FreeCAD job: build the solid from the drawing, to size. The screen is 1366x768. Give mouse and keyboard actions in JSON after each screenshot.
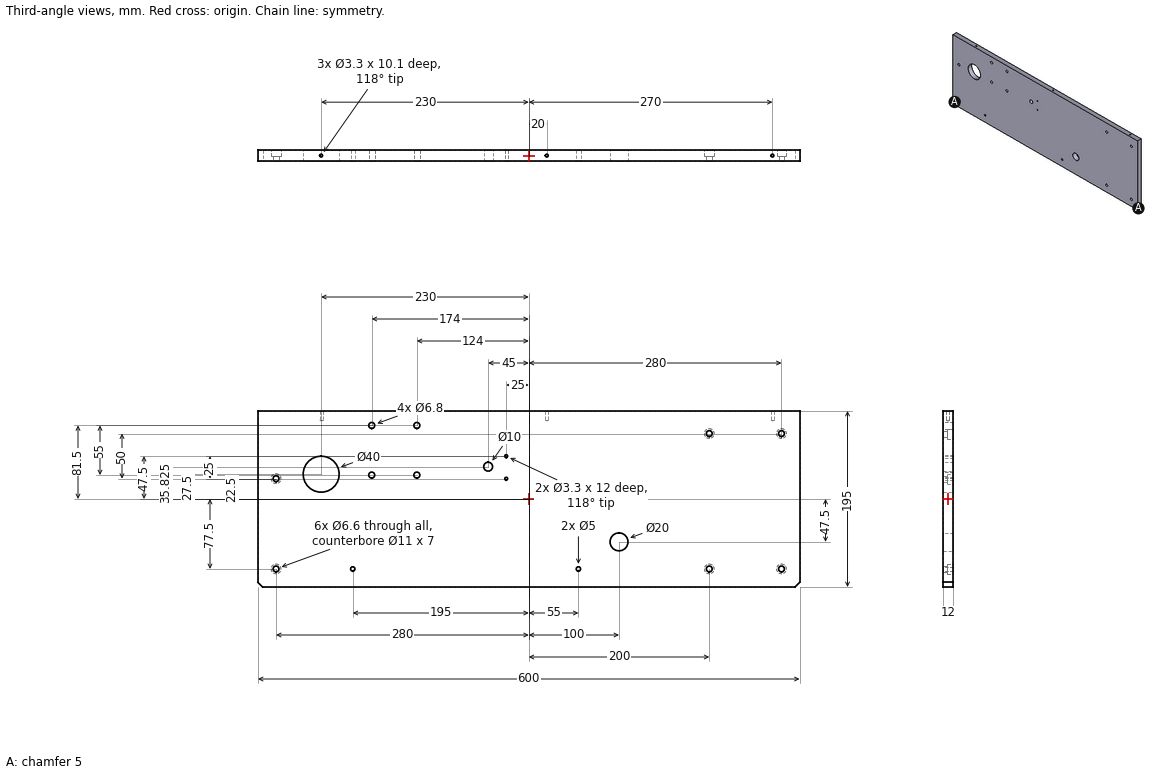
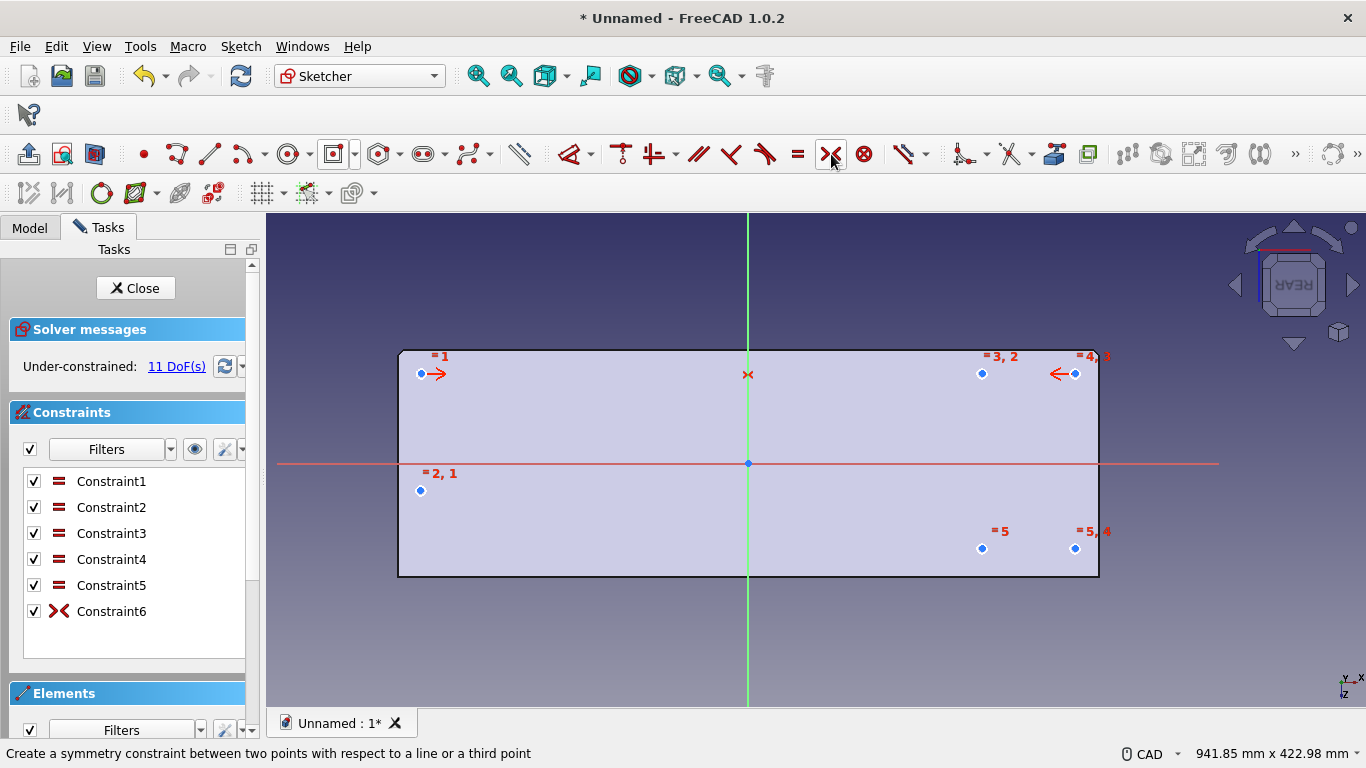
{"action": "key", "text": "d"}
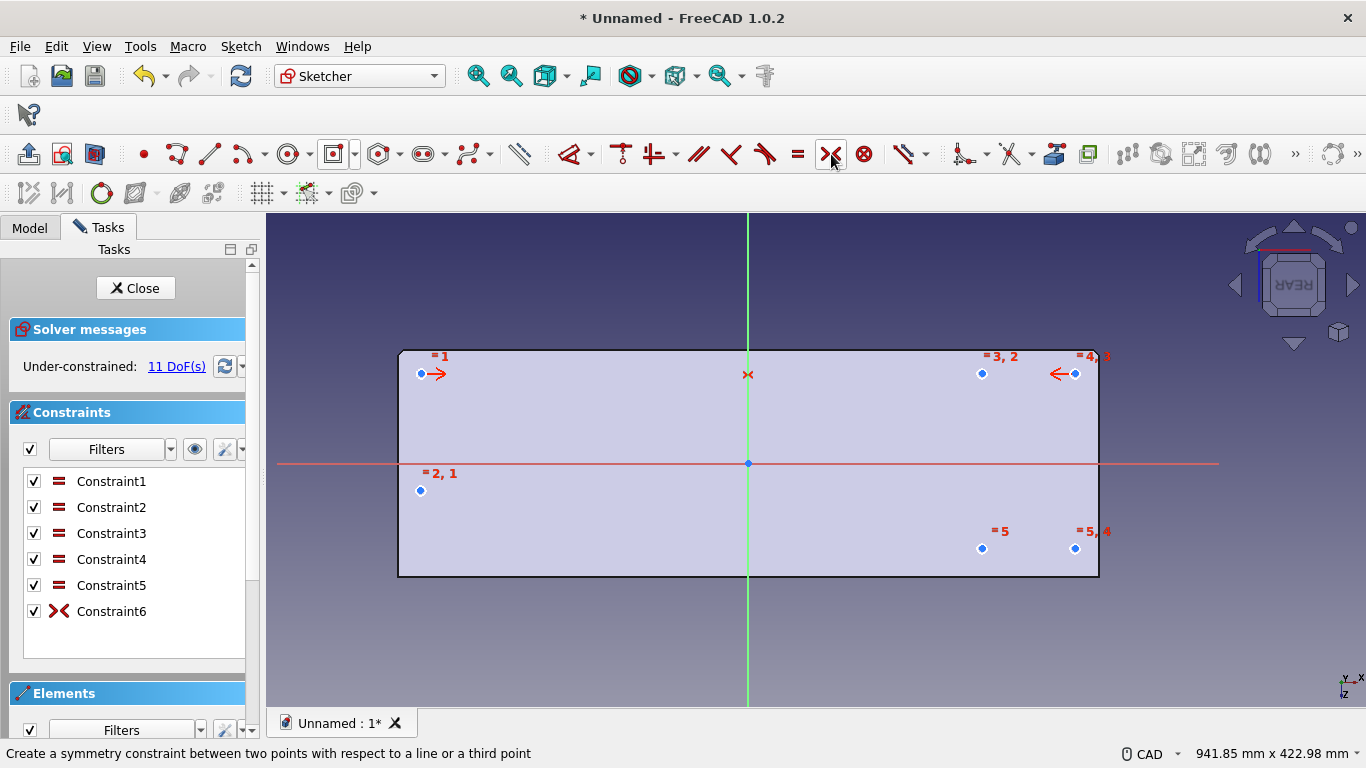
{"action": "scroll", "coordinate": [417, 374], "scroll_direction": "up", "scroll_amount": 9}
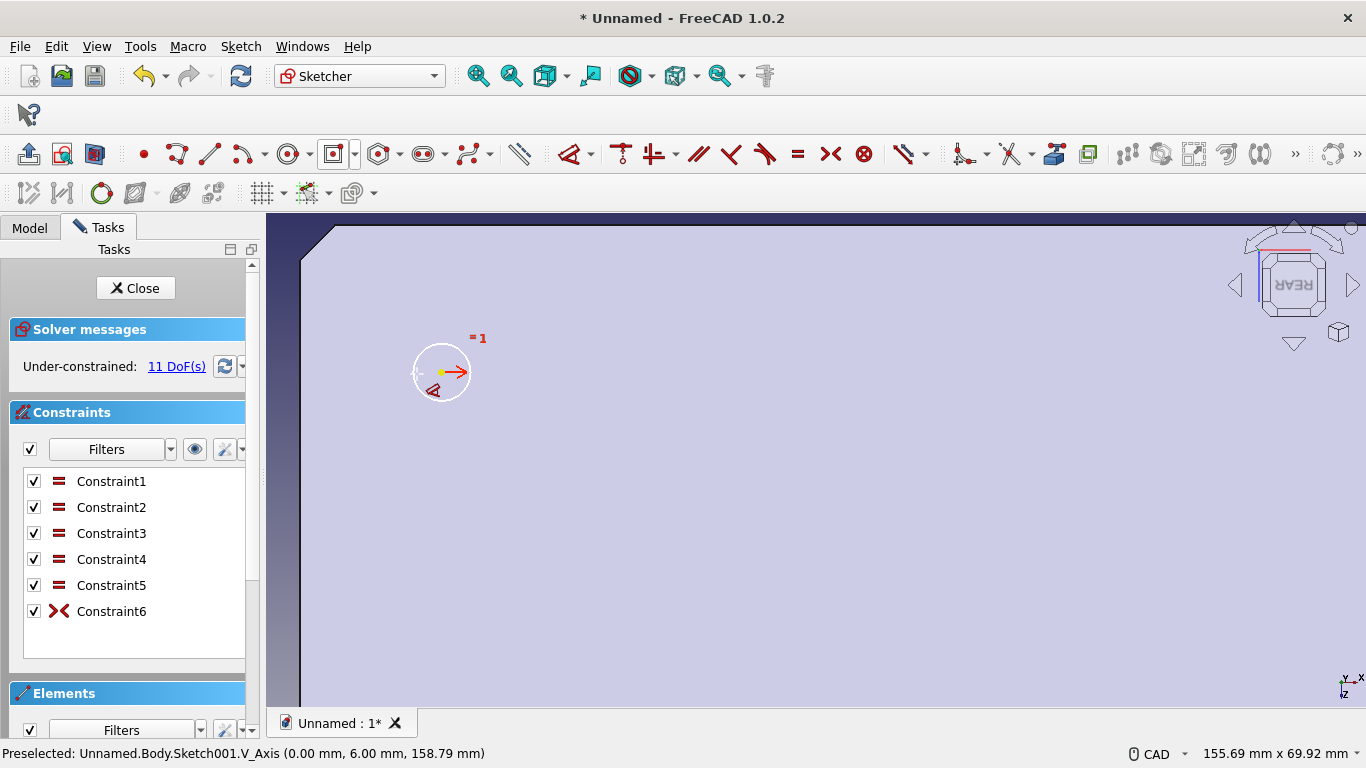
{"action": "left_click", "coordinate": [413, 372]}
{"action": "left_click", "coordinate": [381, 372]}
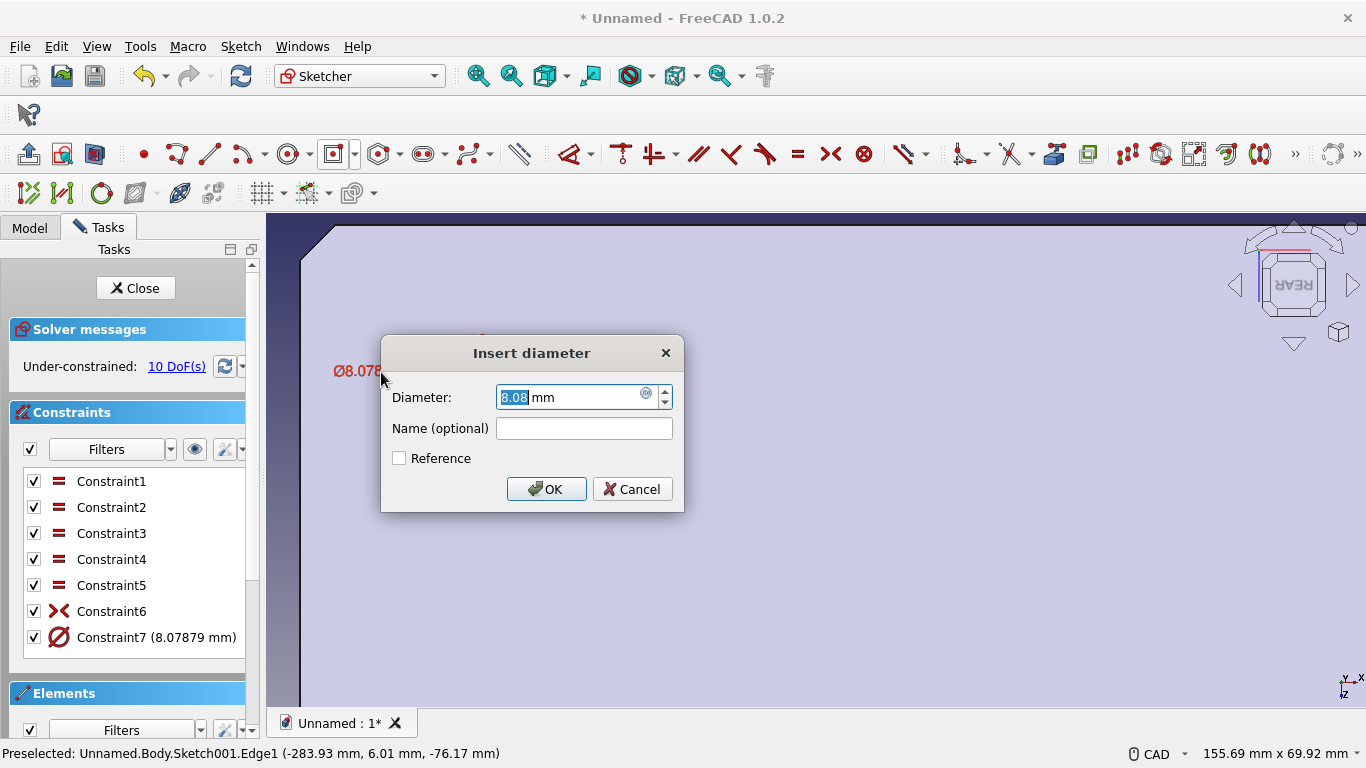
{"action": "type", "text": "6.6"}
{"action": "key", "text": "Return"}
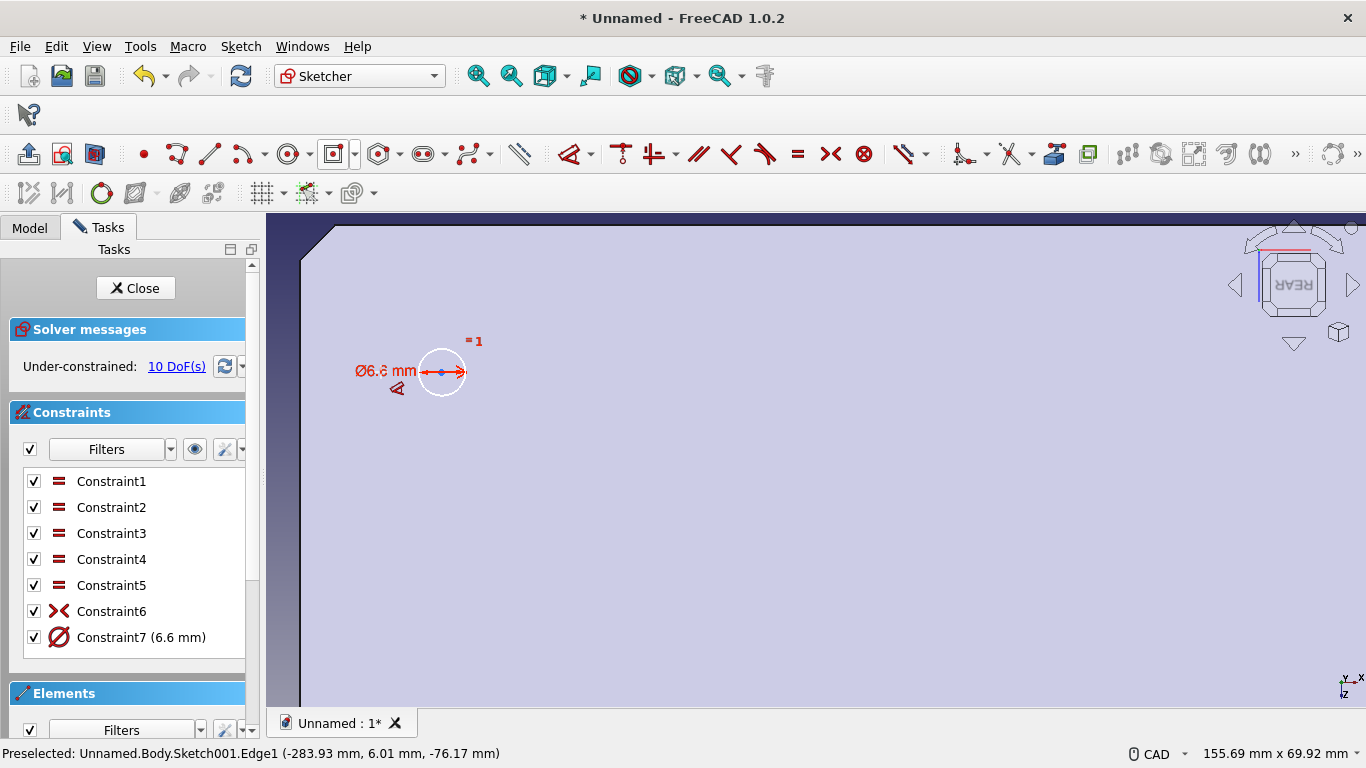
{"action": "scroll", "coordinate": [416, 374], "scroll_direction": "down", "scroll_amount": 9}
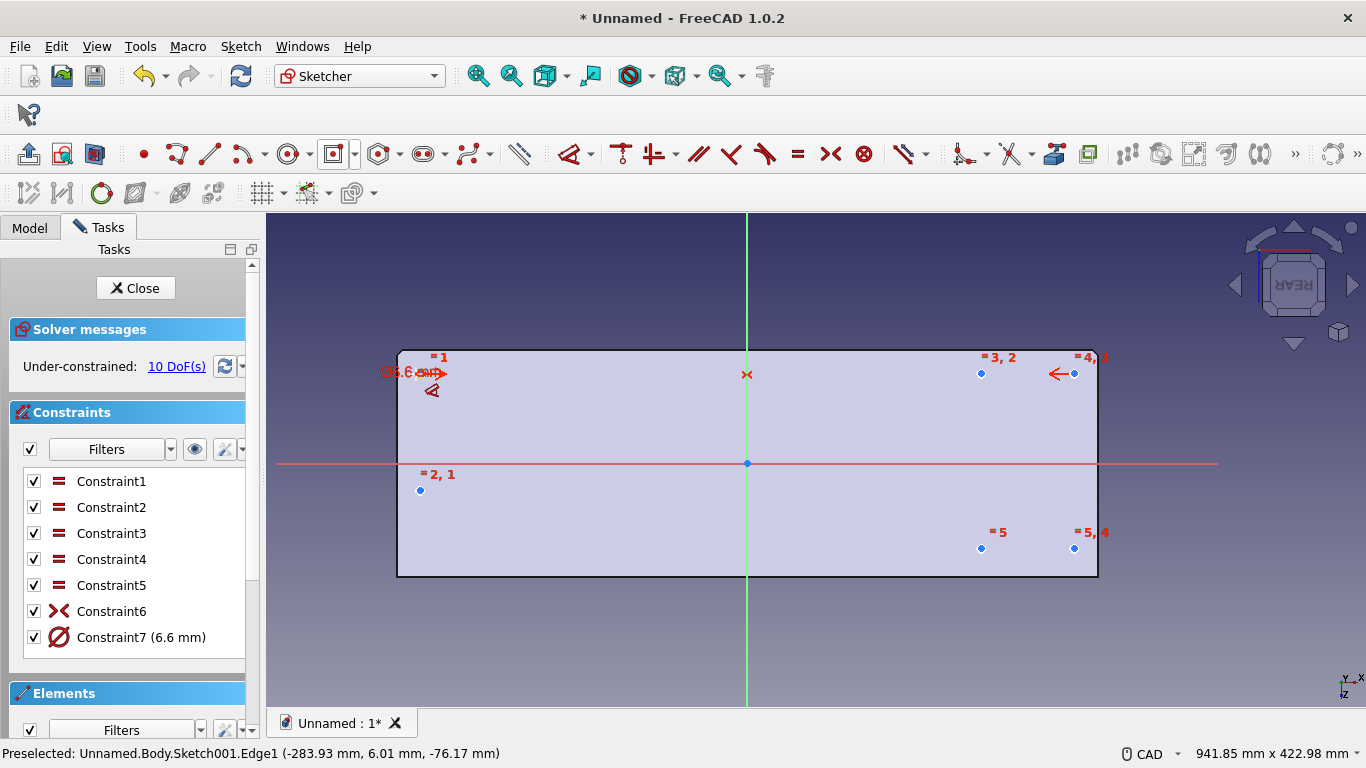
{"action": "left_click", "coordinate": [420, 374]}
{"action": "left_click", "coordinate": [584, 340]}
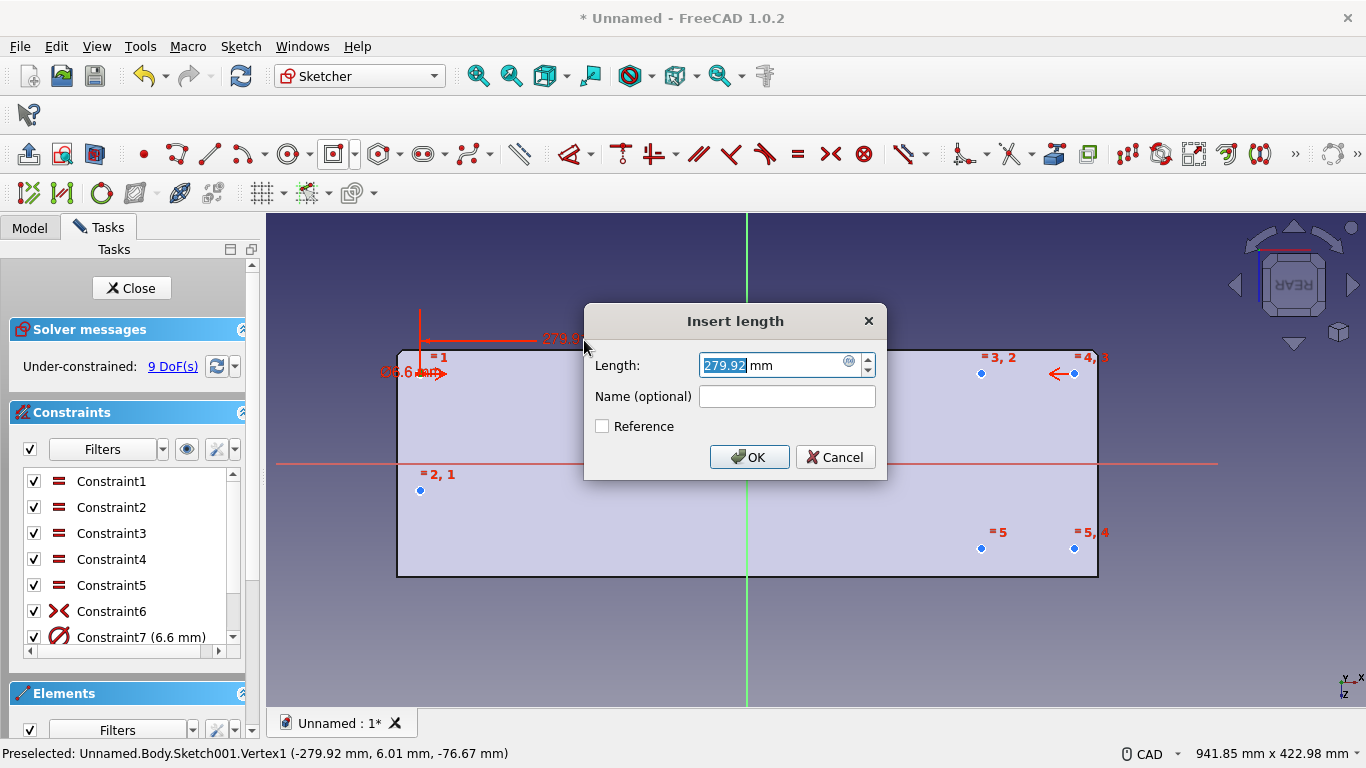
{"action": "type", "text": "280"}
{"action": "key", "text": "Return"}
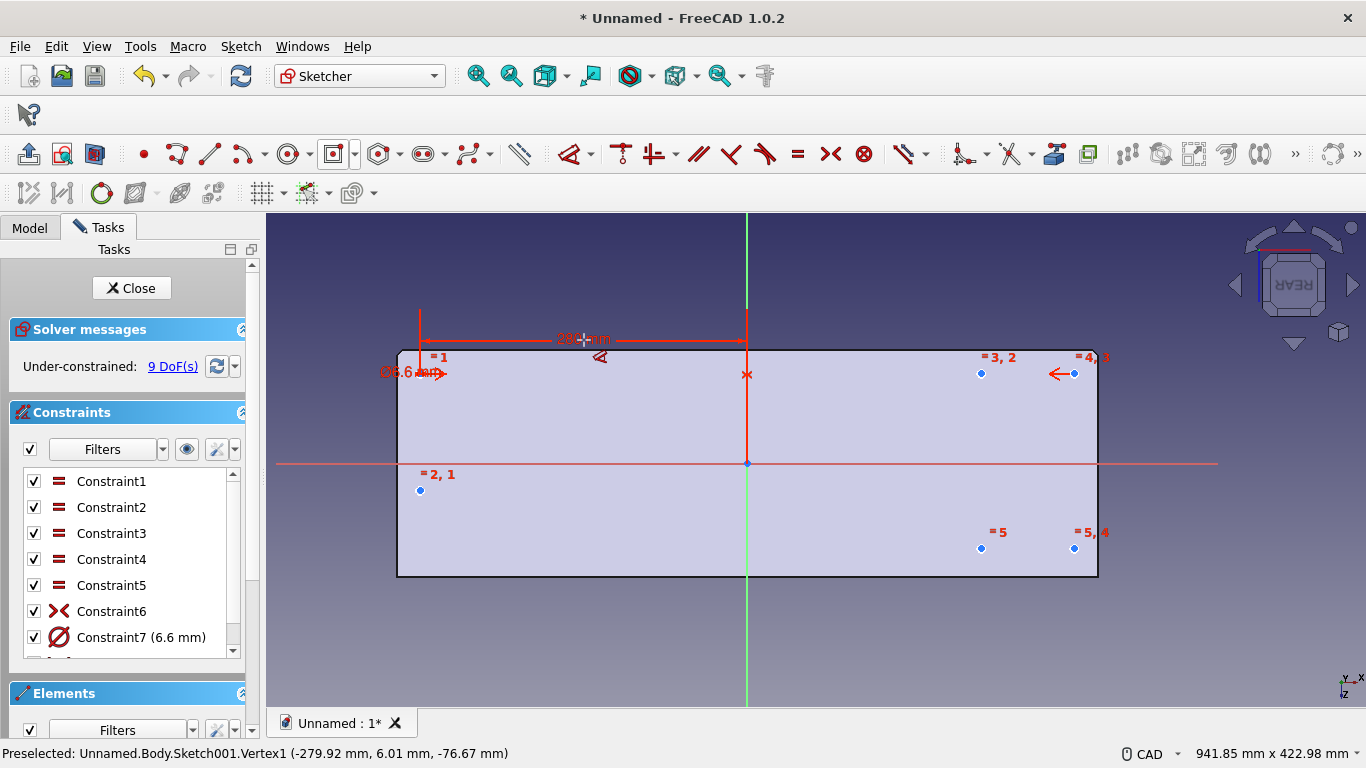
{"action": "left_click", "coordinate": [420, 491]}
{"action": "left_click", "coordinate": [584, 525]}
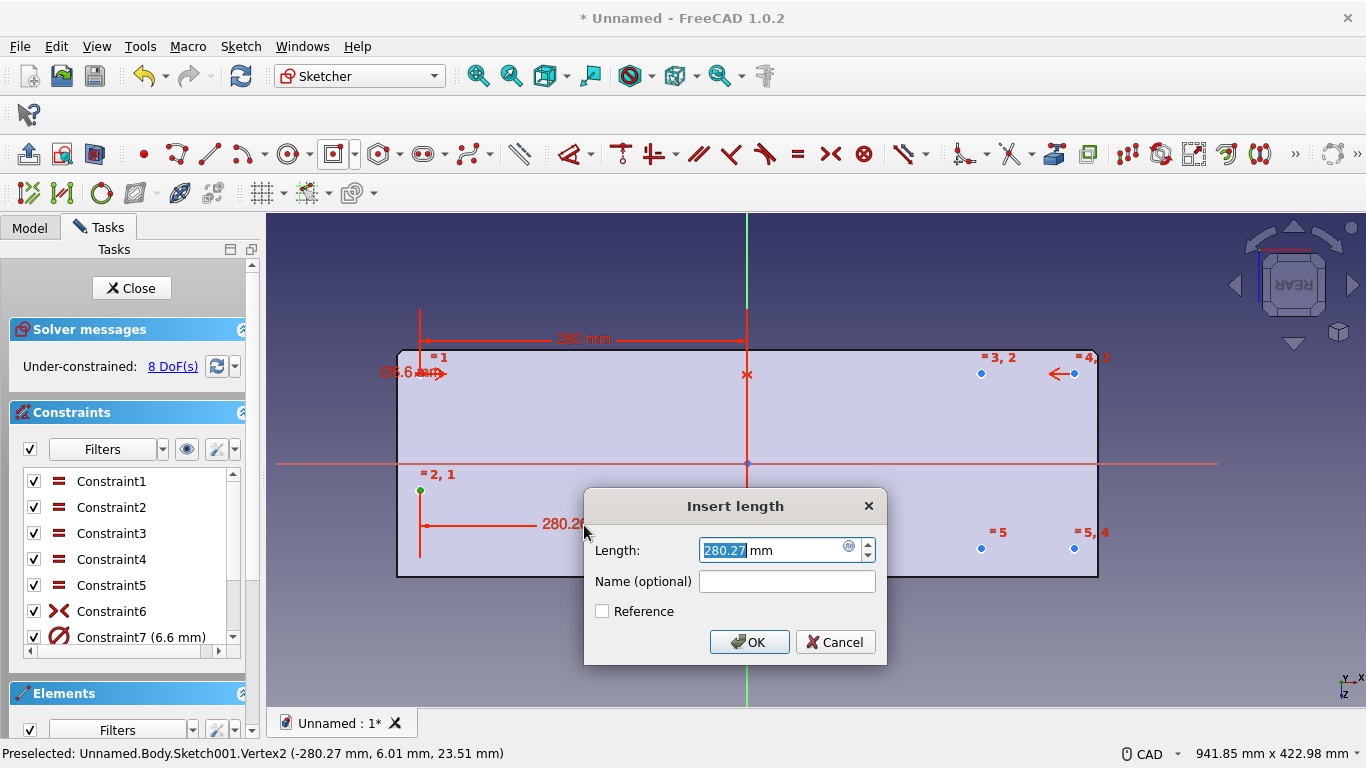
{"action": "type", "text": "280"}
{"action": "key", "text": "Return"}